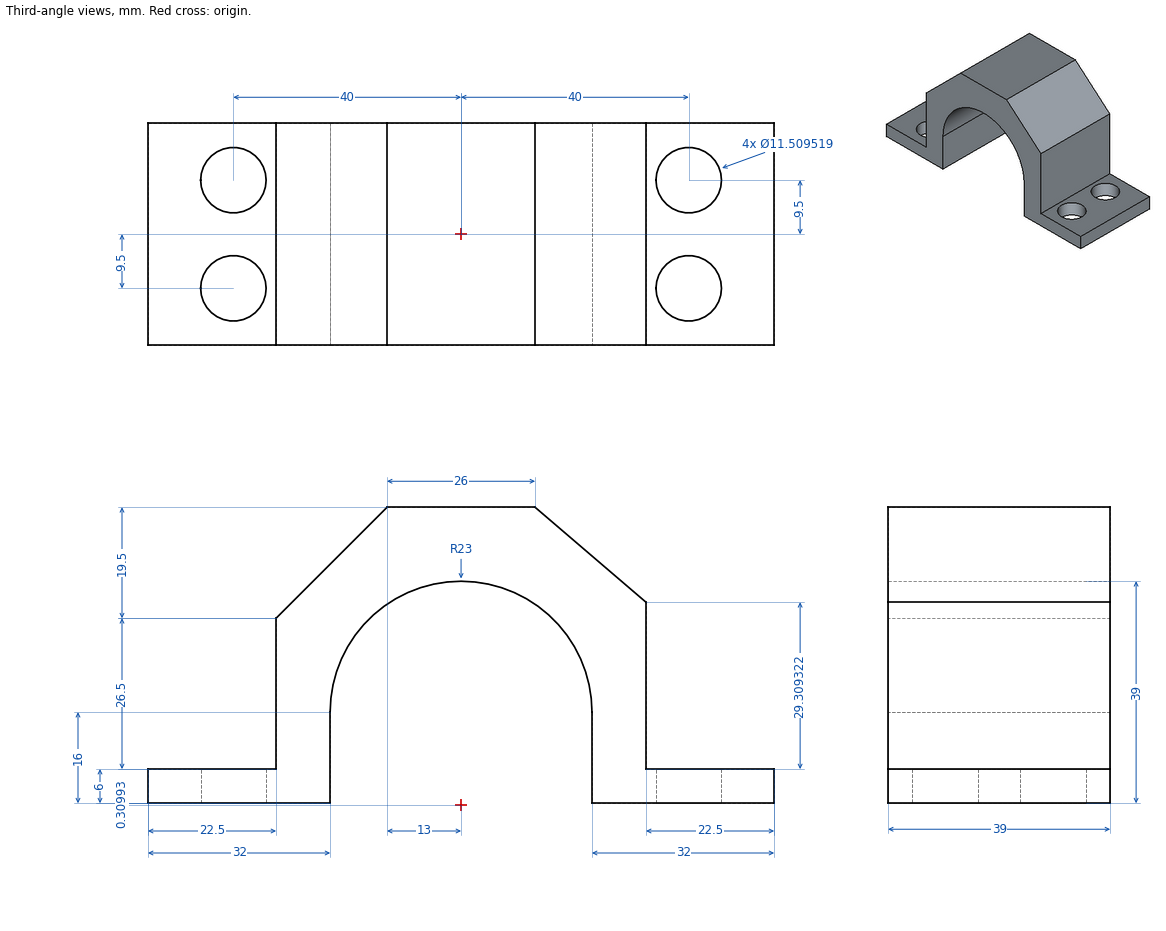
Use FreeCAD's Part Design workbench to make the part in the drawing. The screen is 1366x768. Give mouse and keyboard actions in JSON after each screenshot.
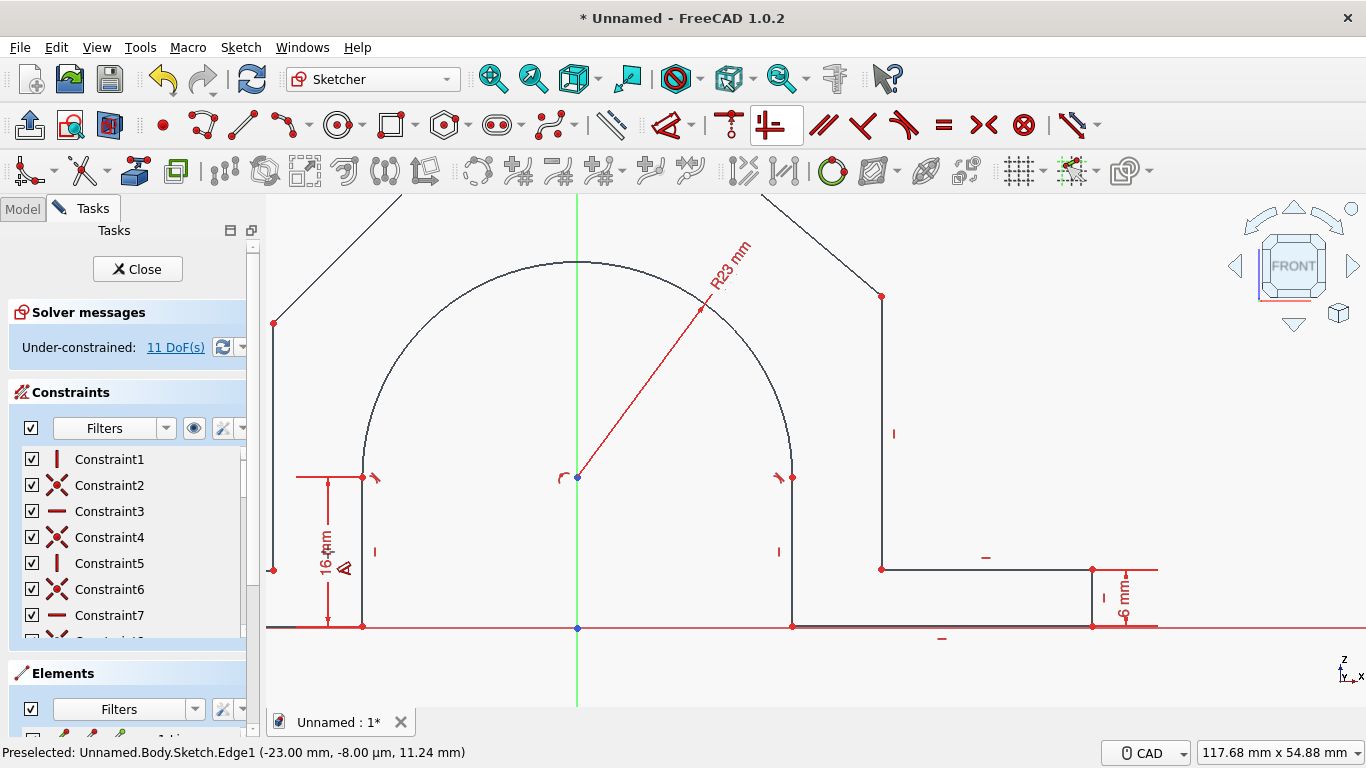
{"action": "left_click", "coordinate": [303, 627]}
{"action": "left_click", "coordinate": [328, 661]}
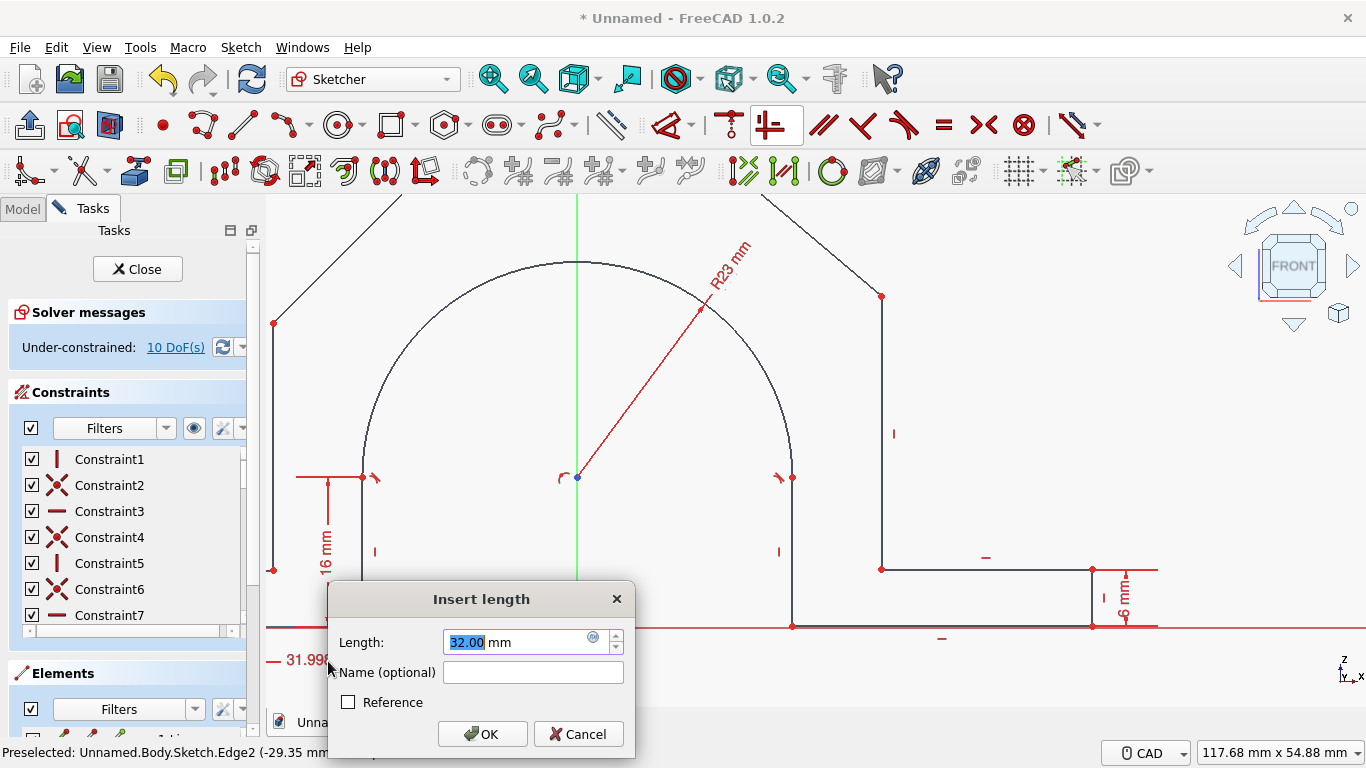
{"action": "type", "text": "32"}
{"action": "key", "text": "Return"}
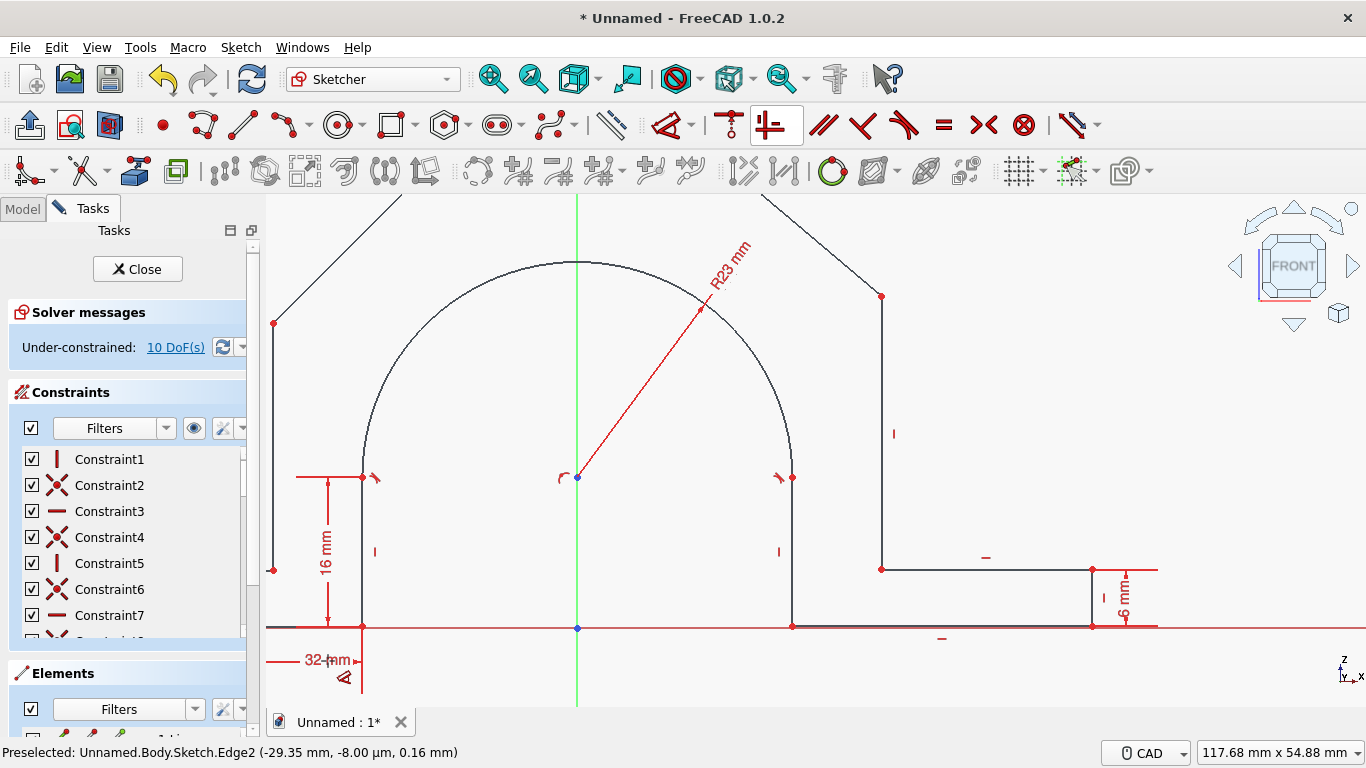
{"action": "scroll", "coordinate": [1093, 587], "scroll_direction": "down", "scroll_amount": 2}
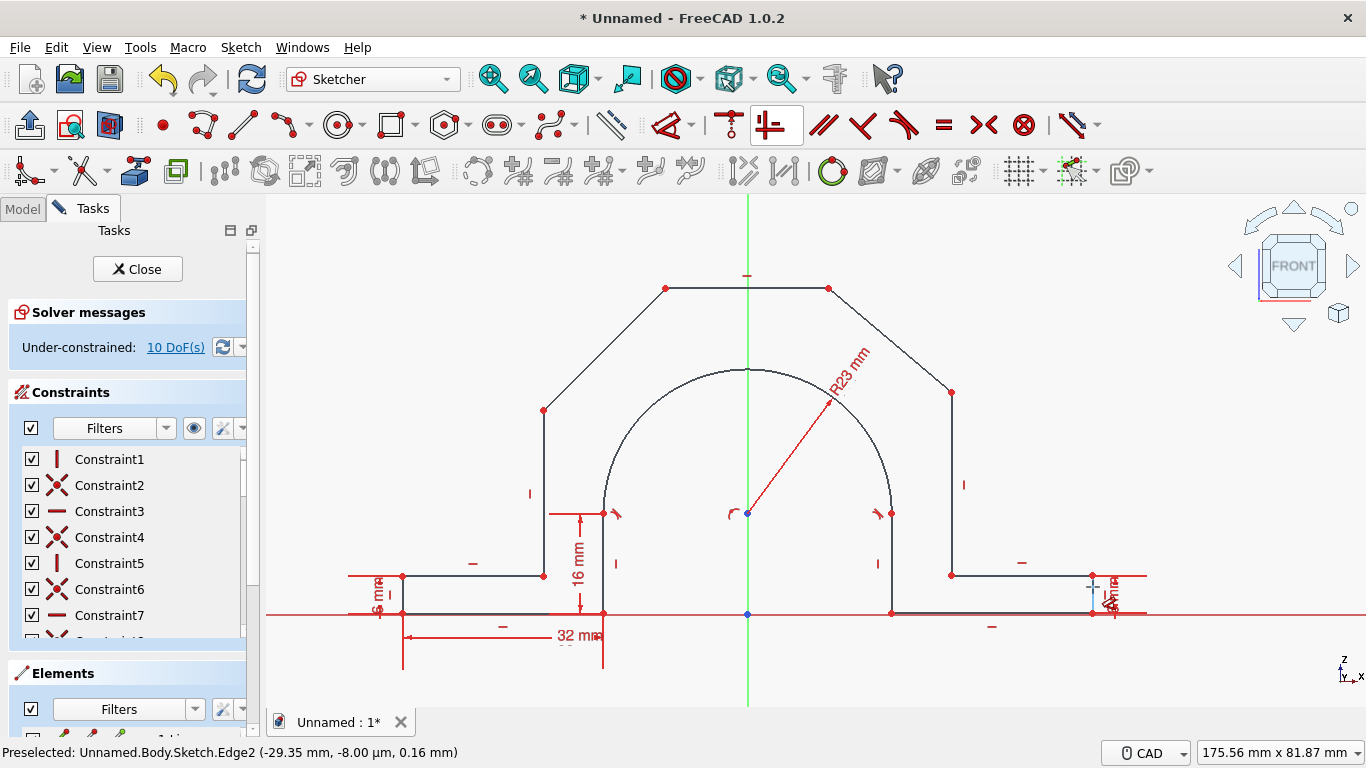
{"action": "left_click", "coordinate": [715, 288]}
{"action": "left_click", "coordinate": [710, 254]}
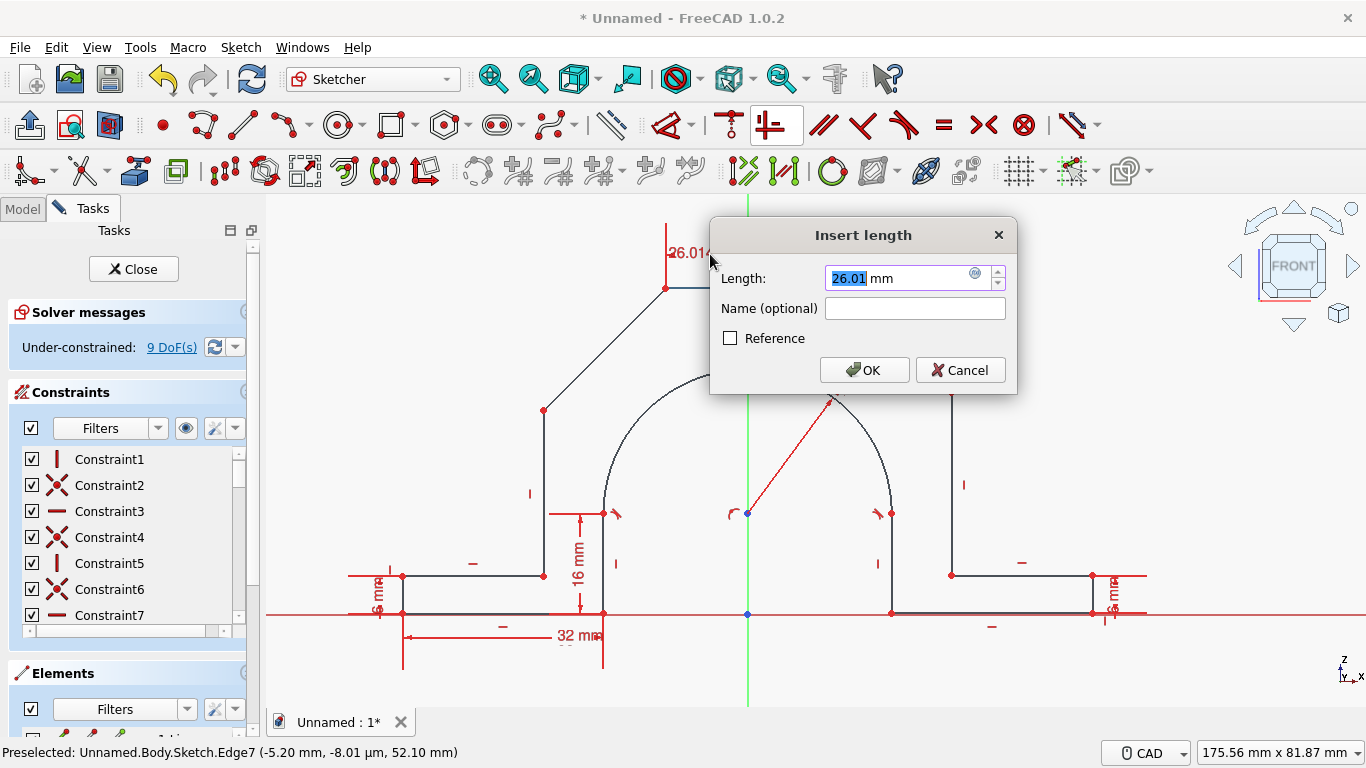
{"action": "type", "text": "26"}
{"action": "key", "text": "Return"}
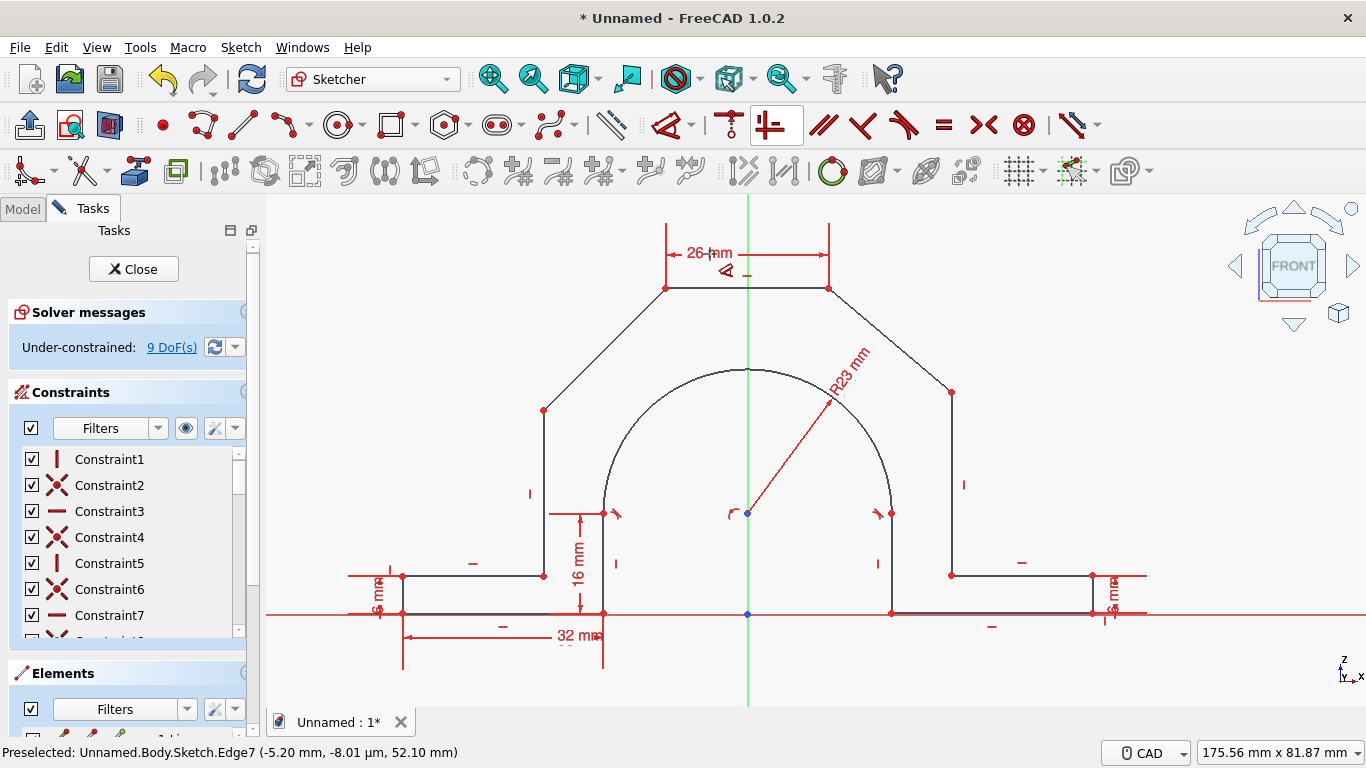
{"action": "left_click", "coordinate": [1032, 613]}
{"action": "left_click", "coordinate": [992, 647]}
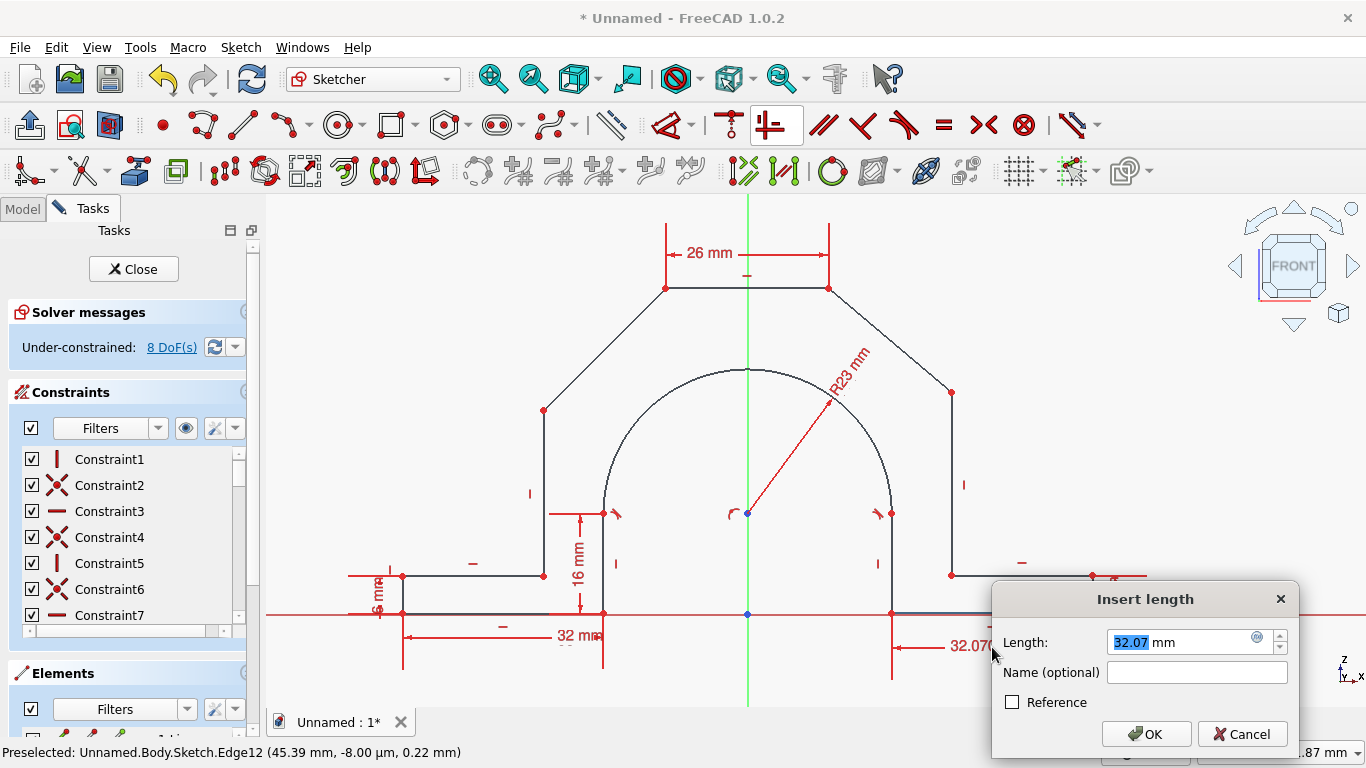
{"action": "type", "text": "32"}
{"action": "key", "text": "Return"}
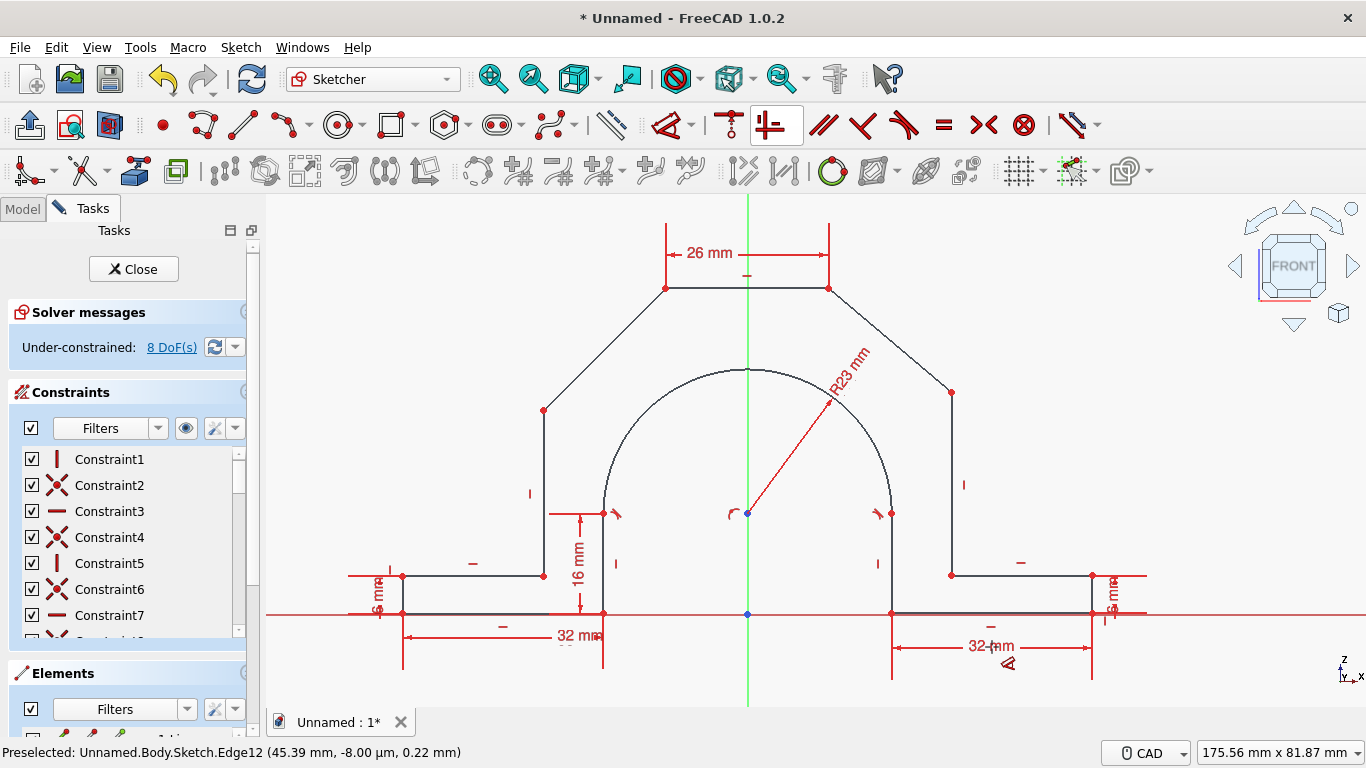
{"action": "left_click", "coordinate": [892, 583]}
{"action": "left_click", "coordinate": [926, 563]}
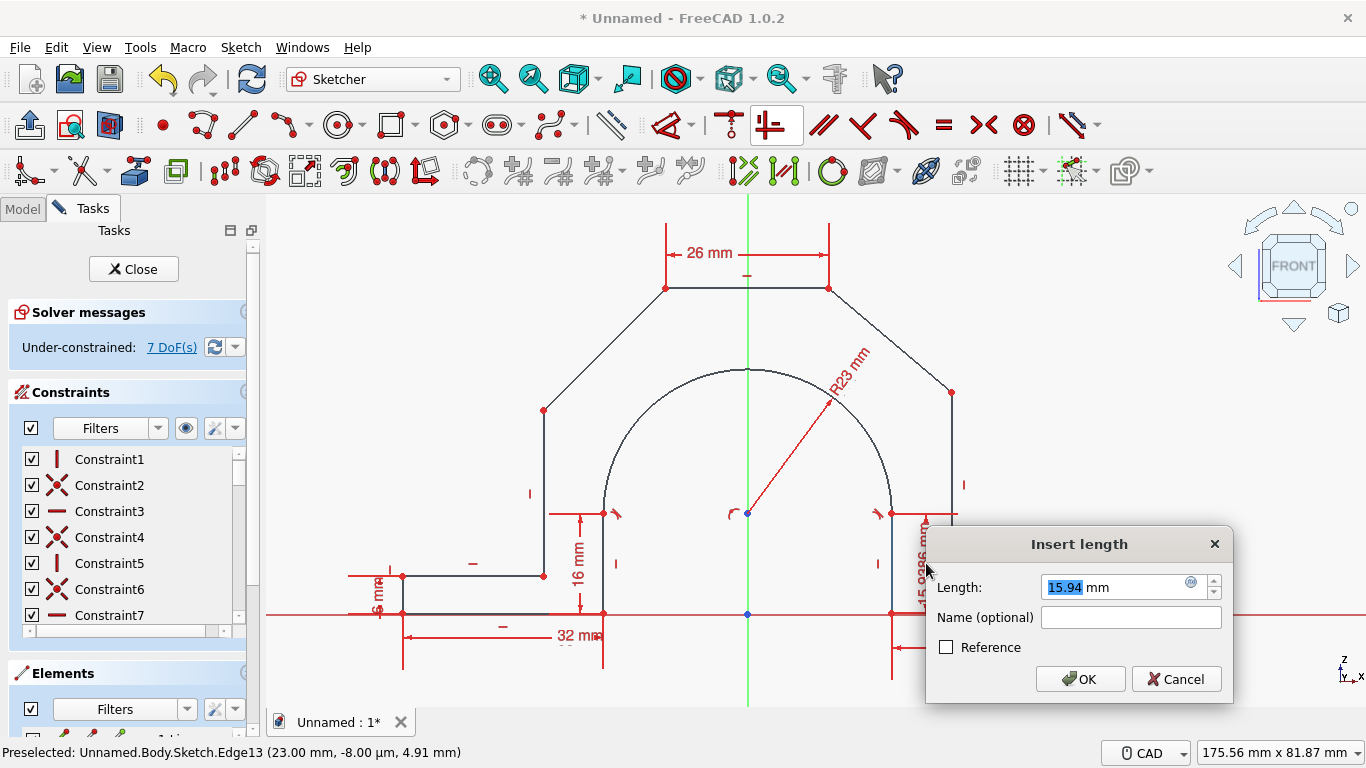
{"action": "type", "text": "16"}
{"action": "key", "text": "Return"}